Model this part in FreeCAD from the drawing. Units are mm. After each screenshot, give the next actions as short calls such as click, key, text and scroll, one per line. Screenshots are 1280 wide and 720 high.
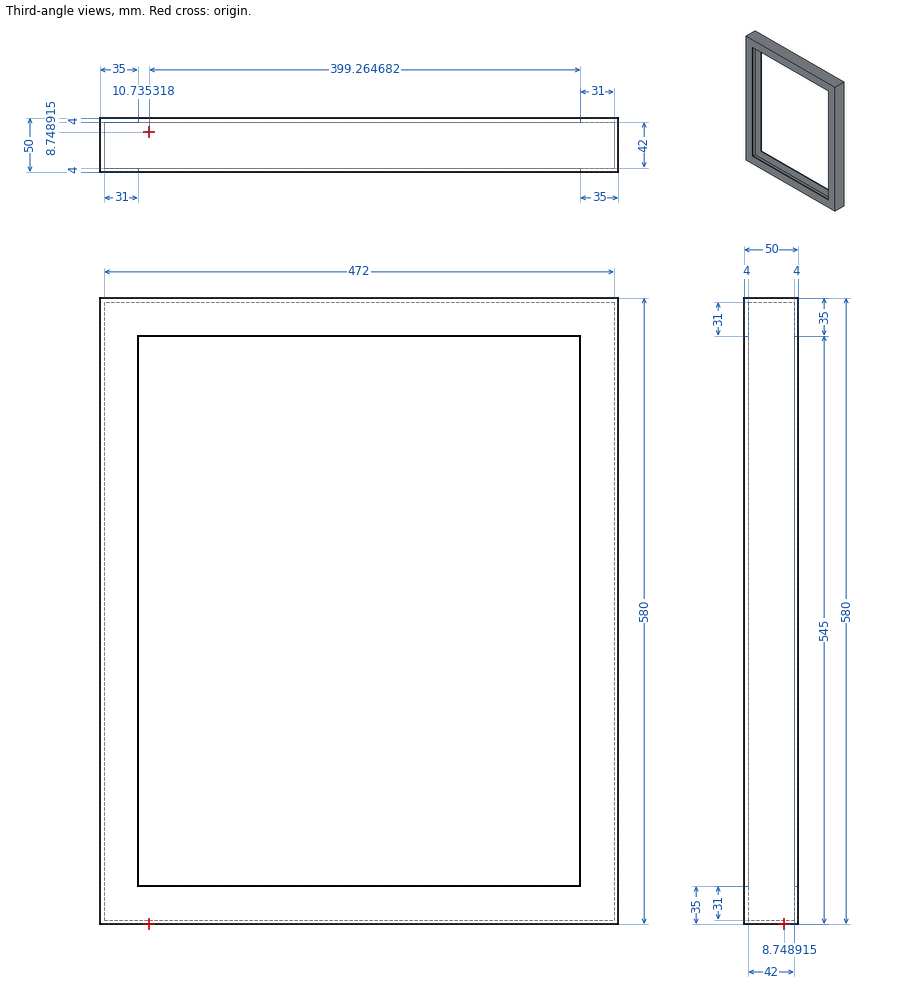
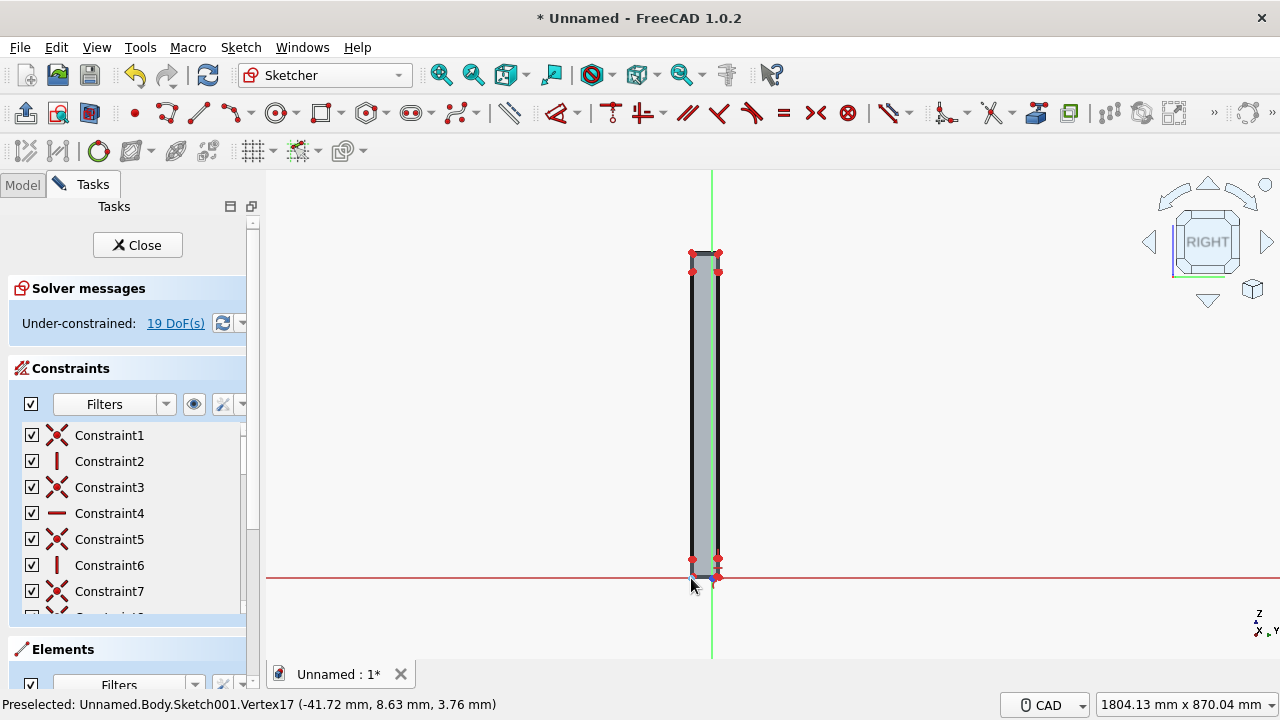
scroll(718, 272, up, 13)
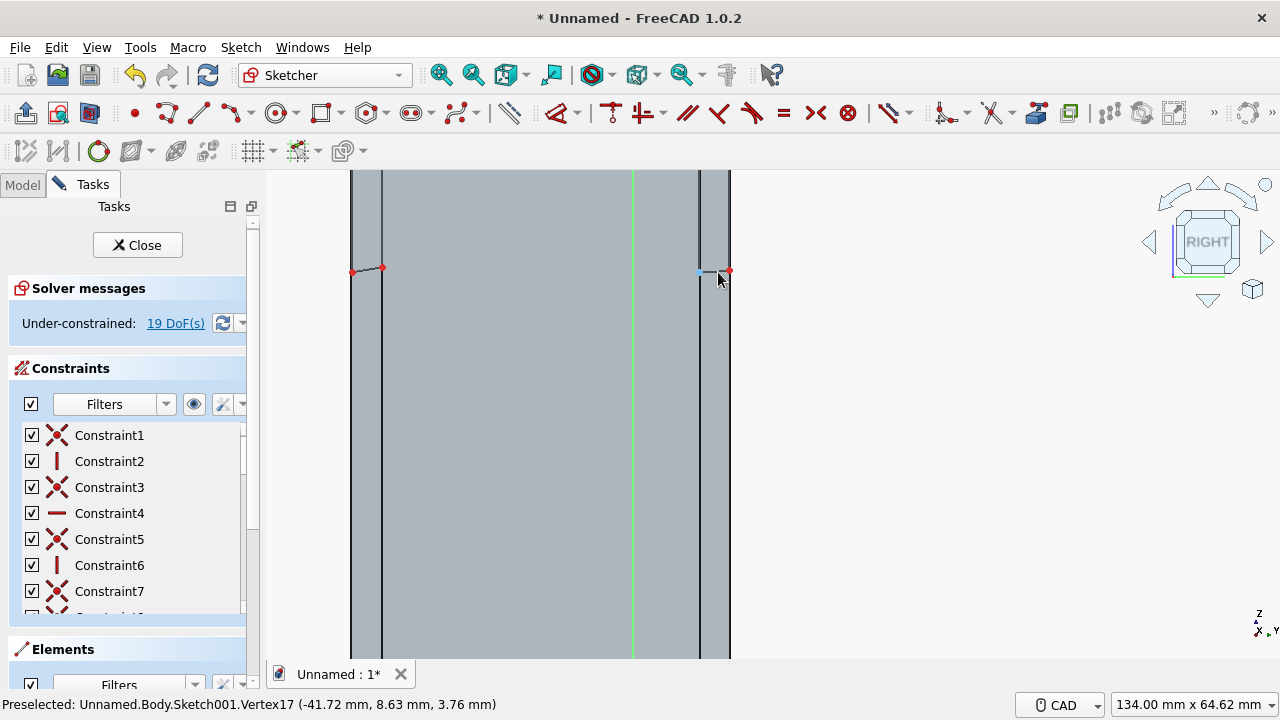
click(714, 272)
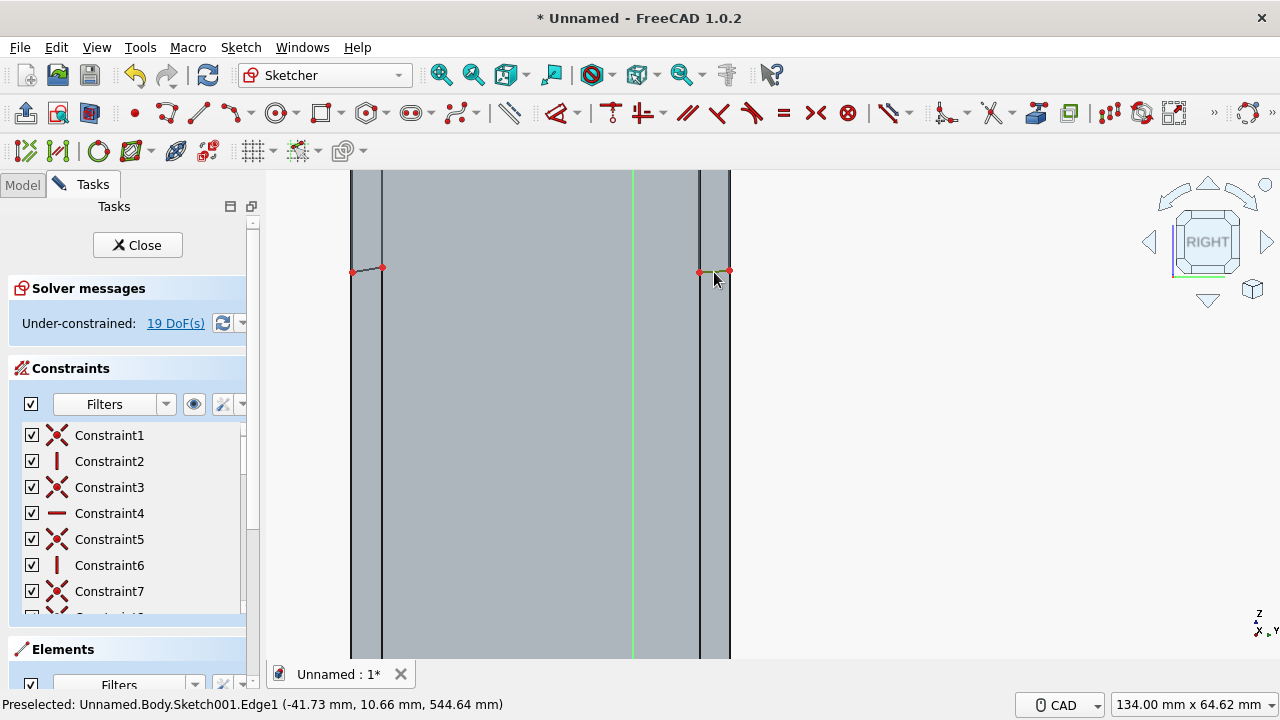
key(h)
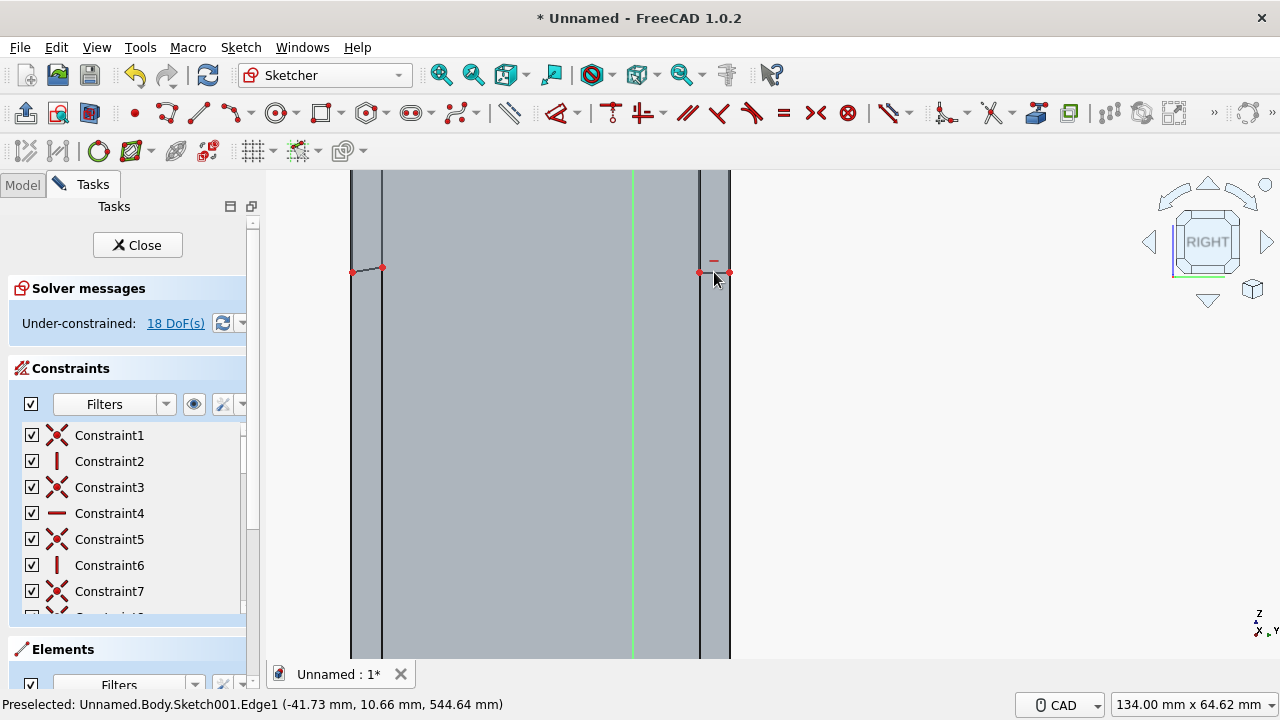
click(361, 271)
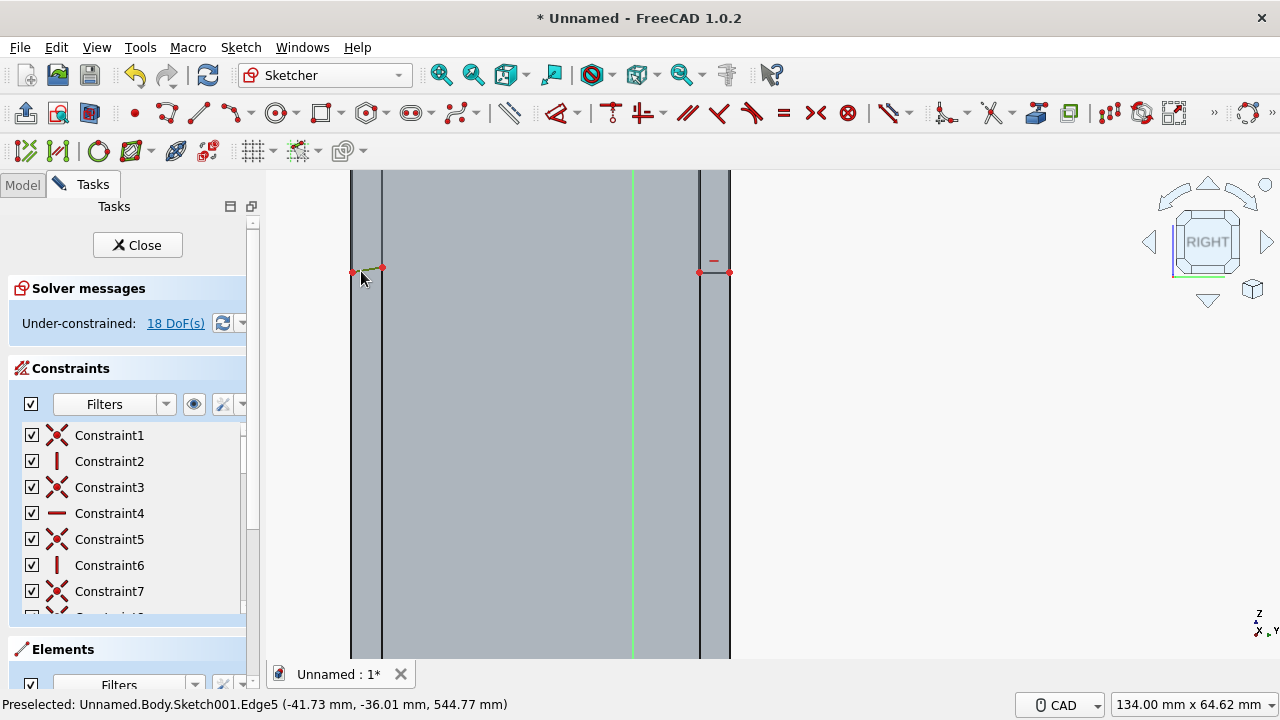
click(666, 114)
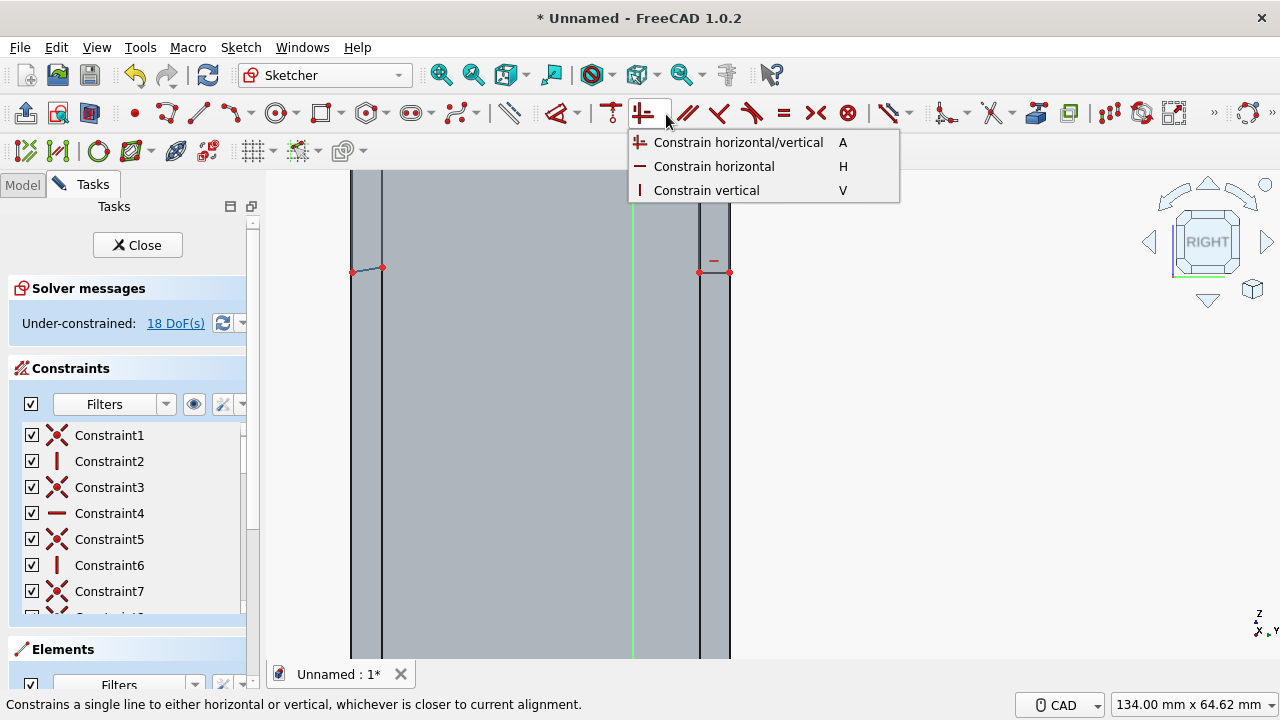
click(764, 166)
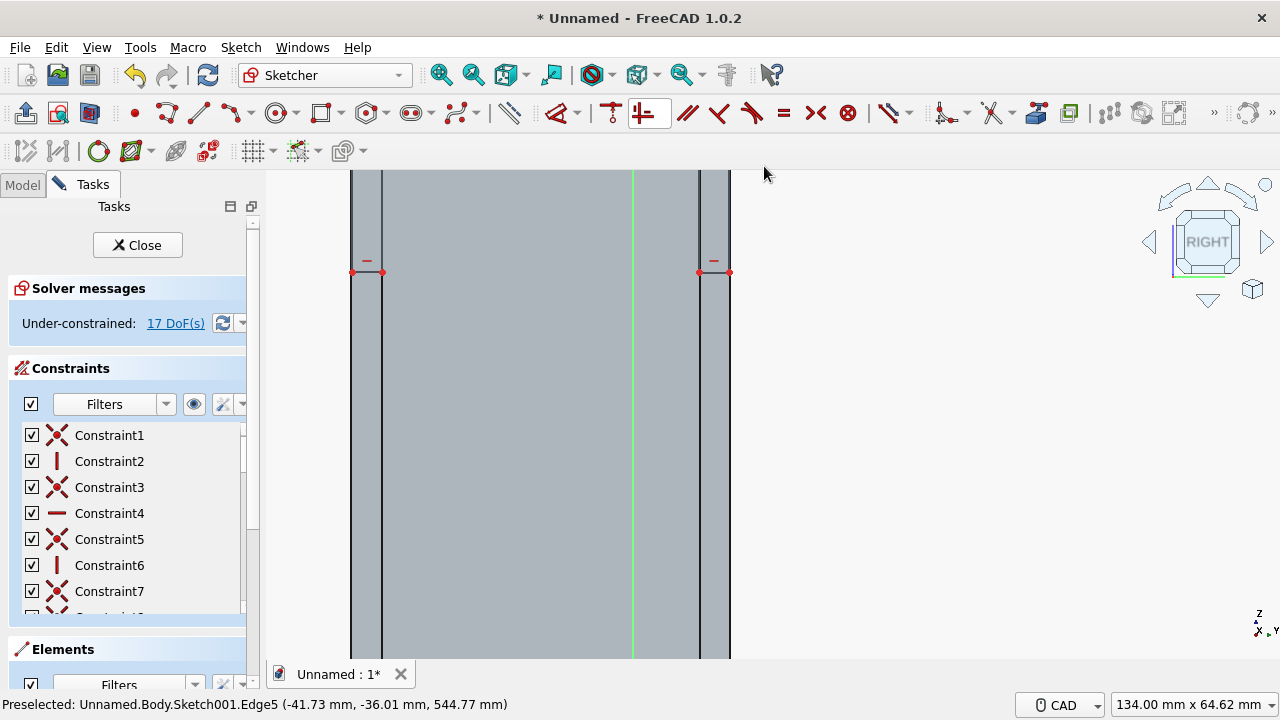
scroll(718, 271, down, 13)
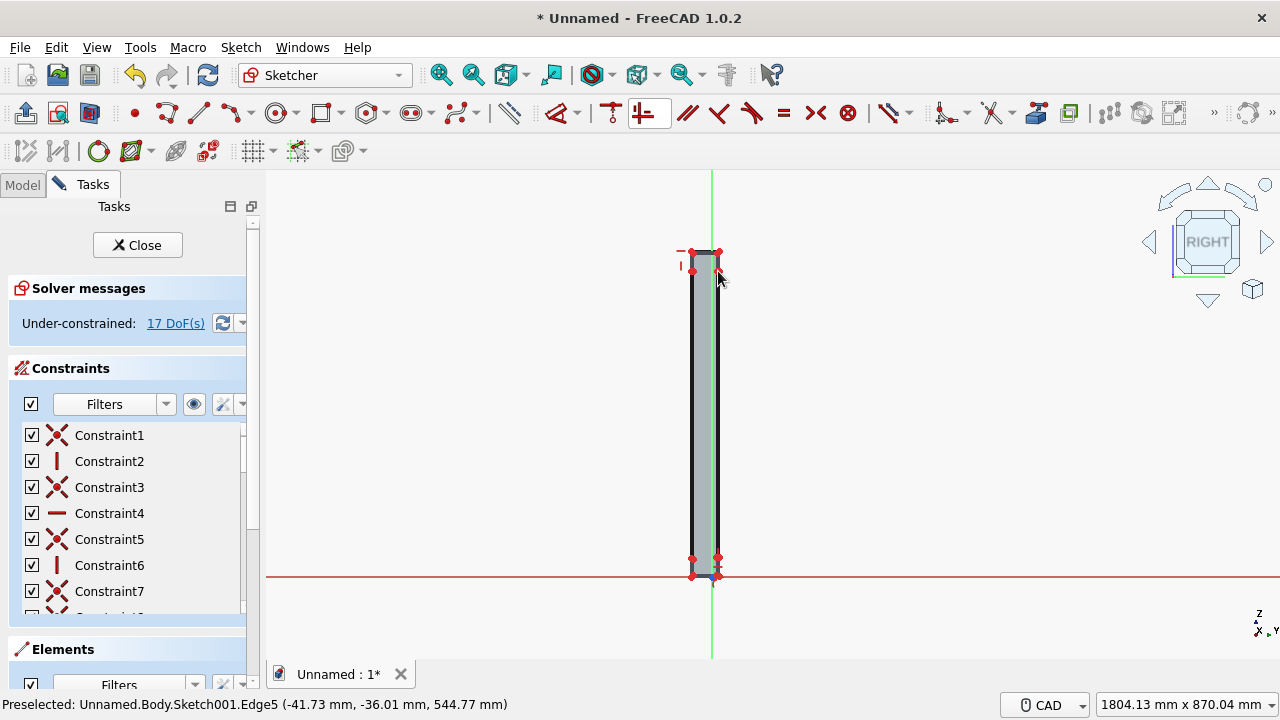
scroll(693, 559, up, 14)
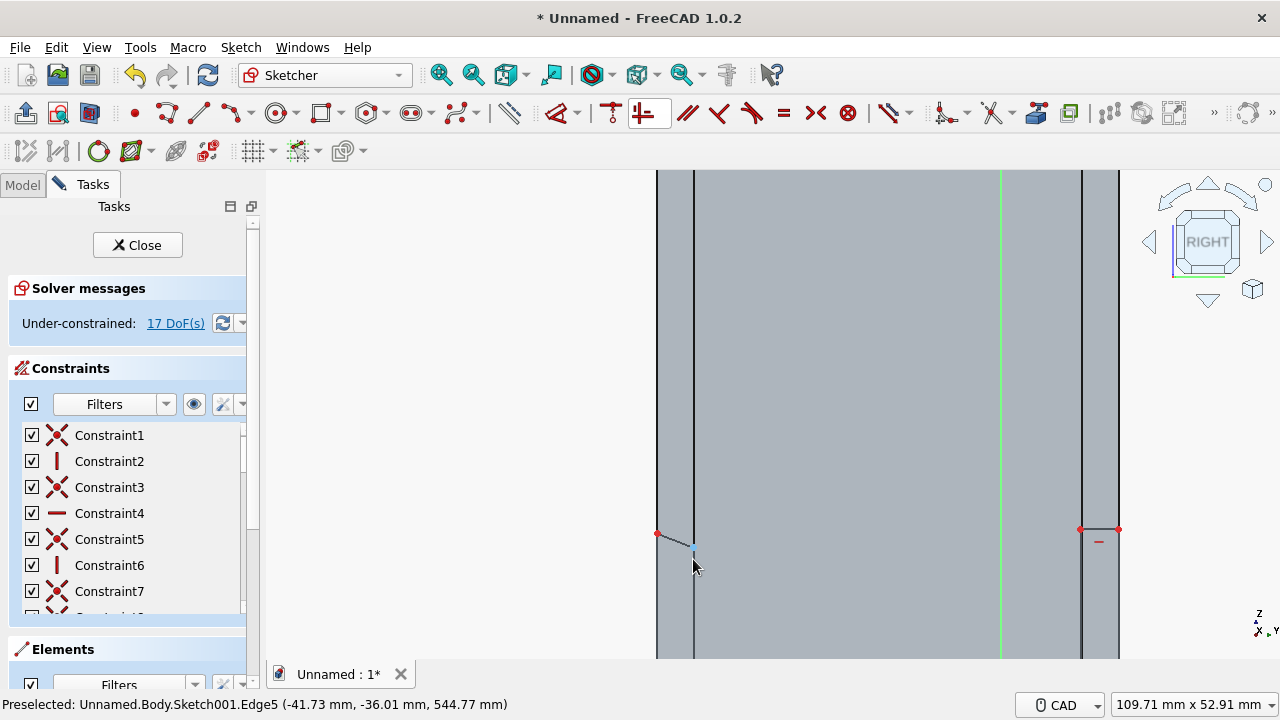
click(683, 544)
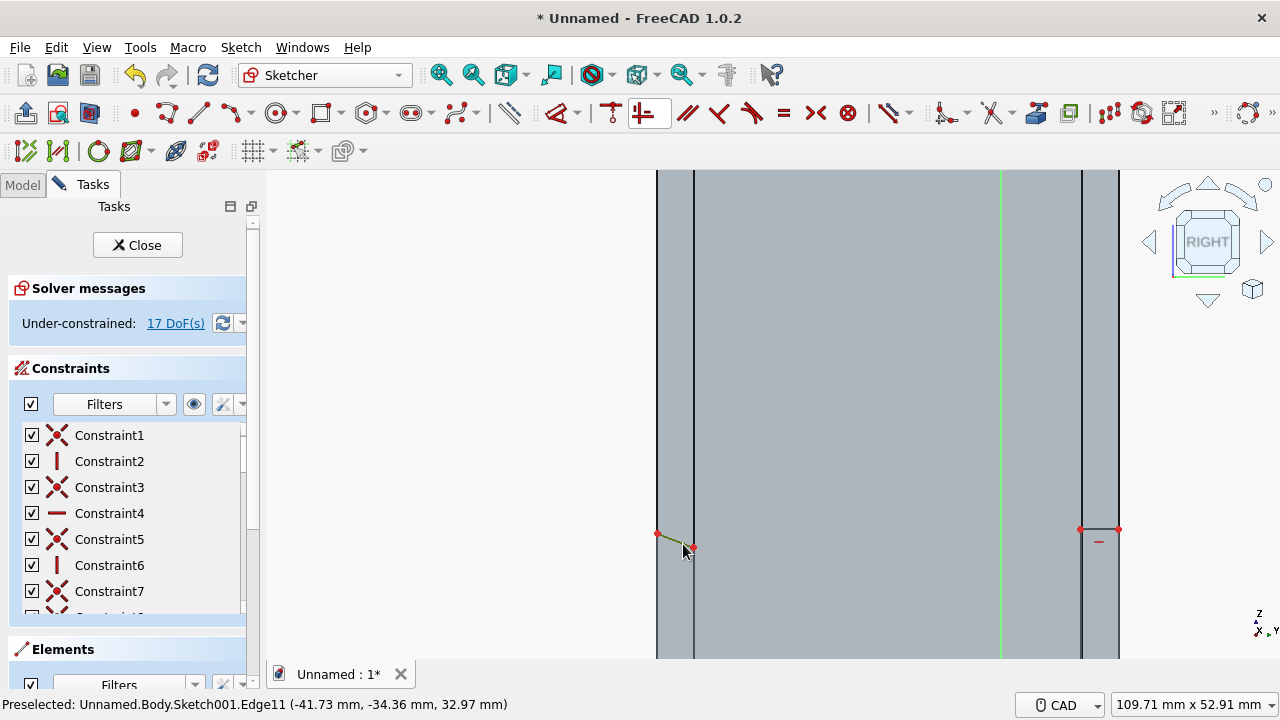
key(h)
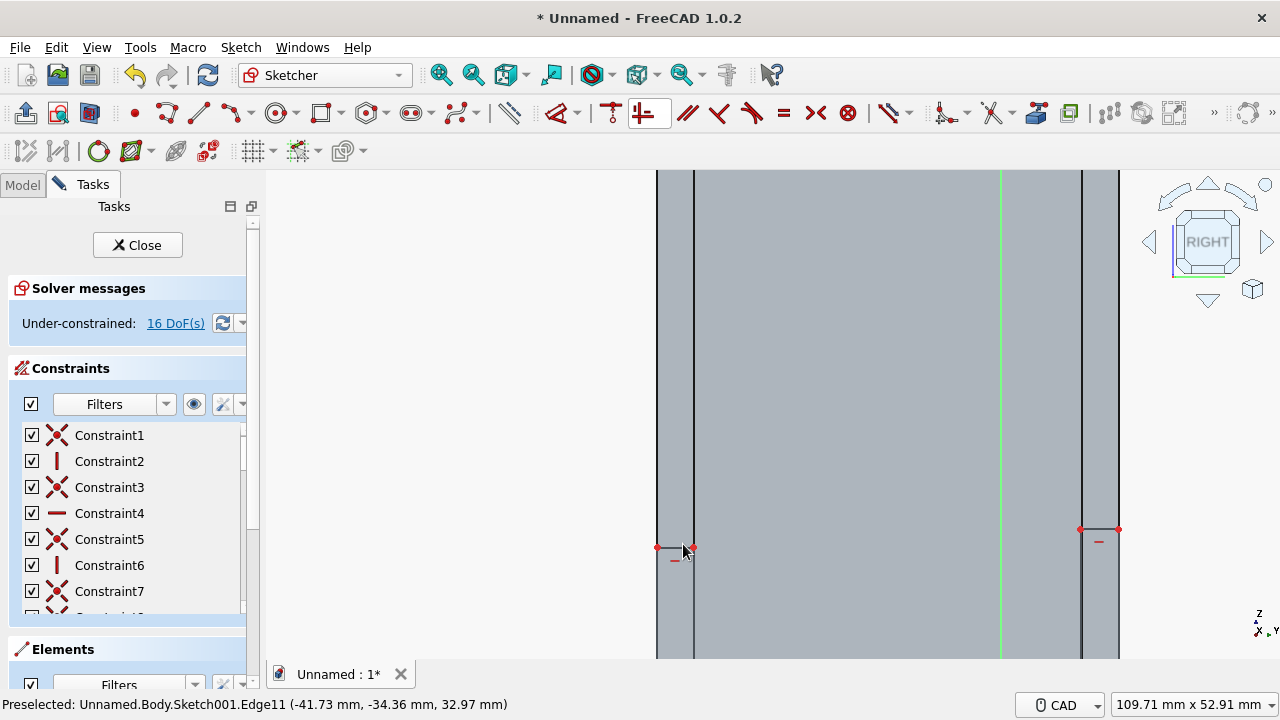
scroll(693, 560, down, 14)